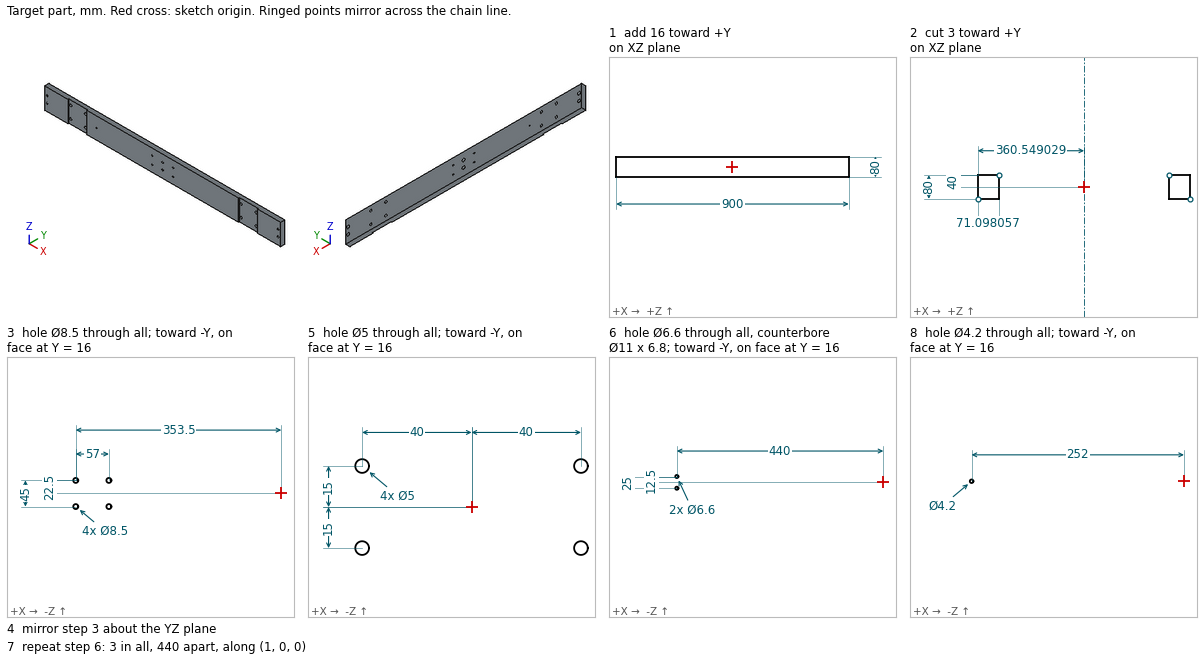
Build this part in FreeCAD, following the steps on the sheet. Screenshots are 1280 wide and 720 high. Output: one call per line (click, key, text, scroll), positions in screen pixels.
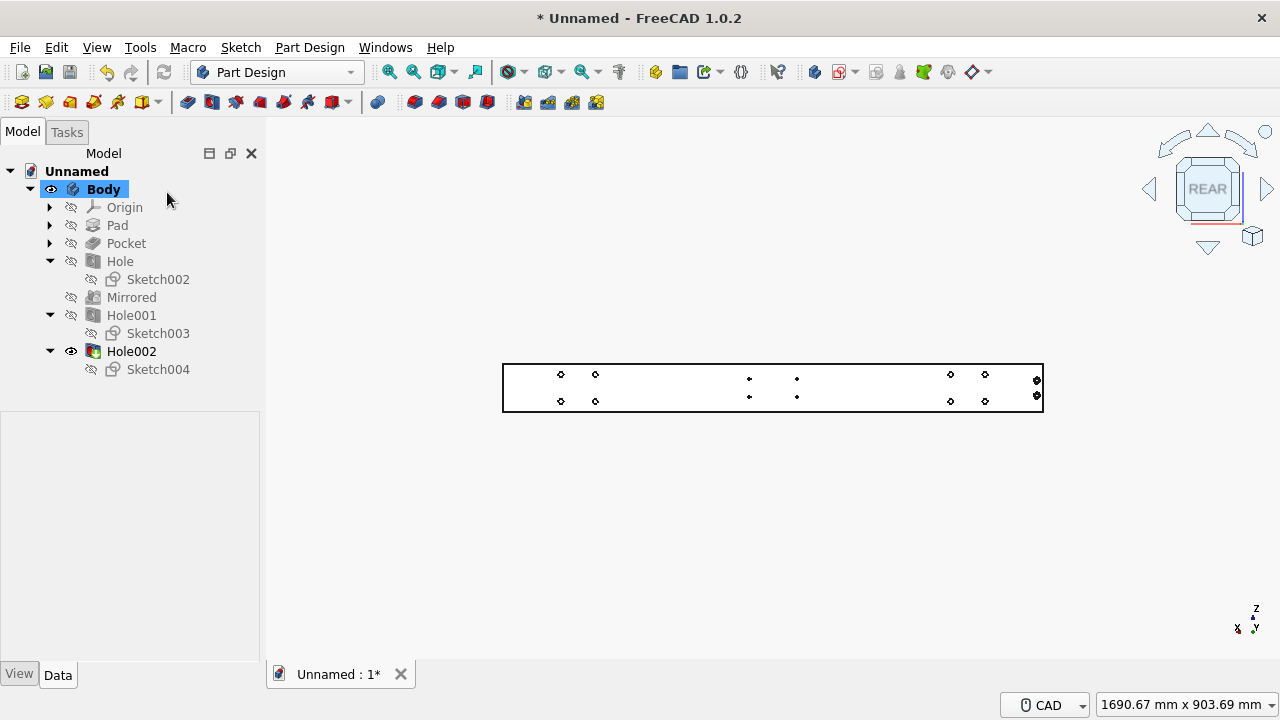
click(116, 351)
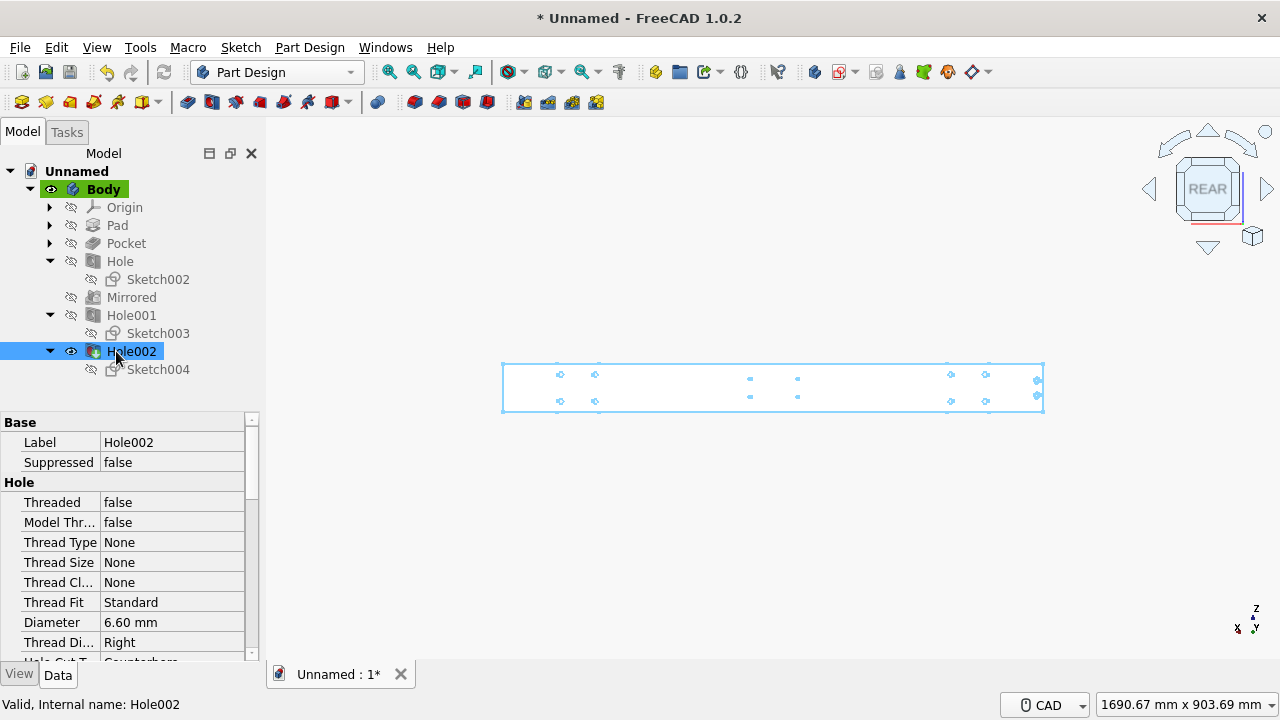
click(548, 102)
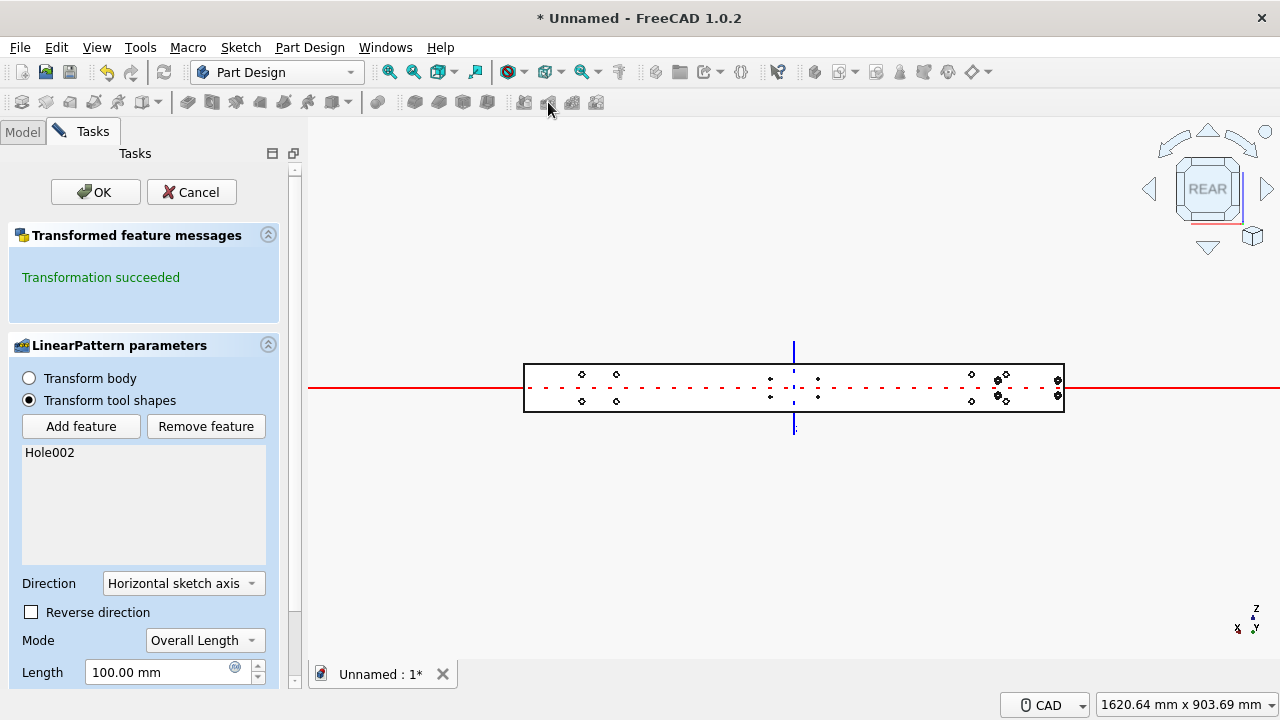
click(184, 584)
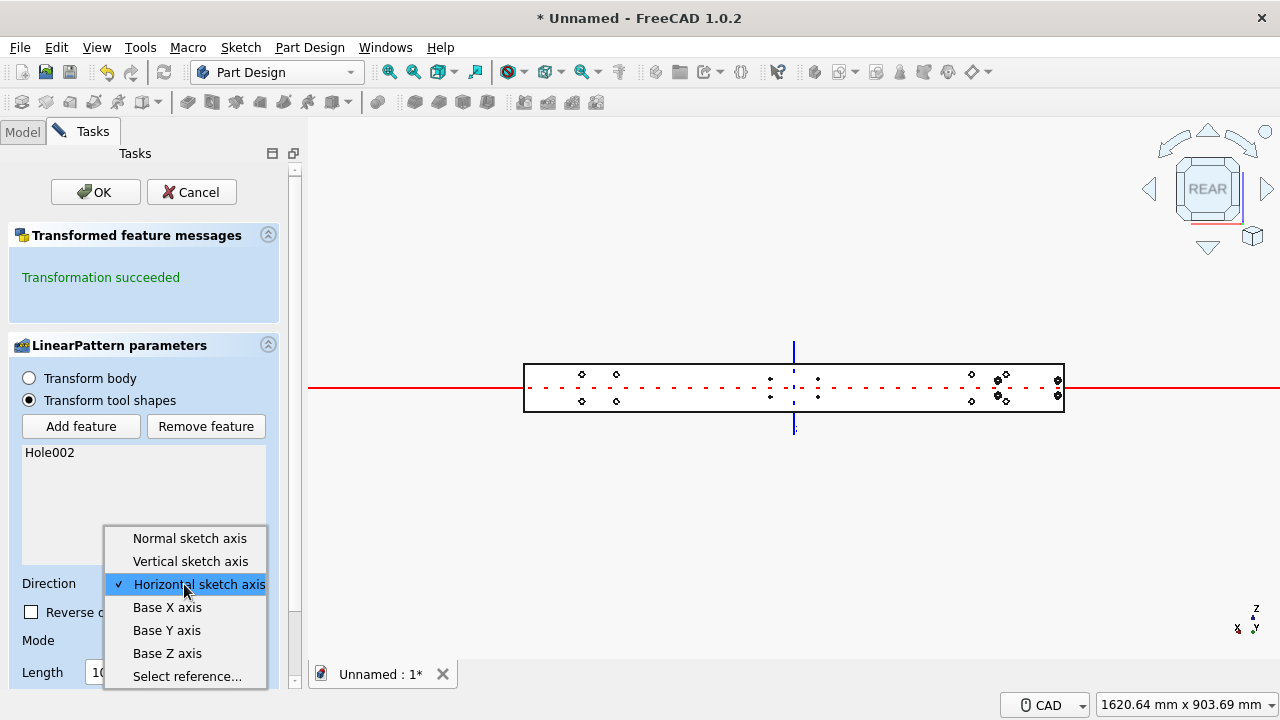
click(184, 608)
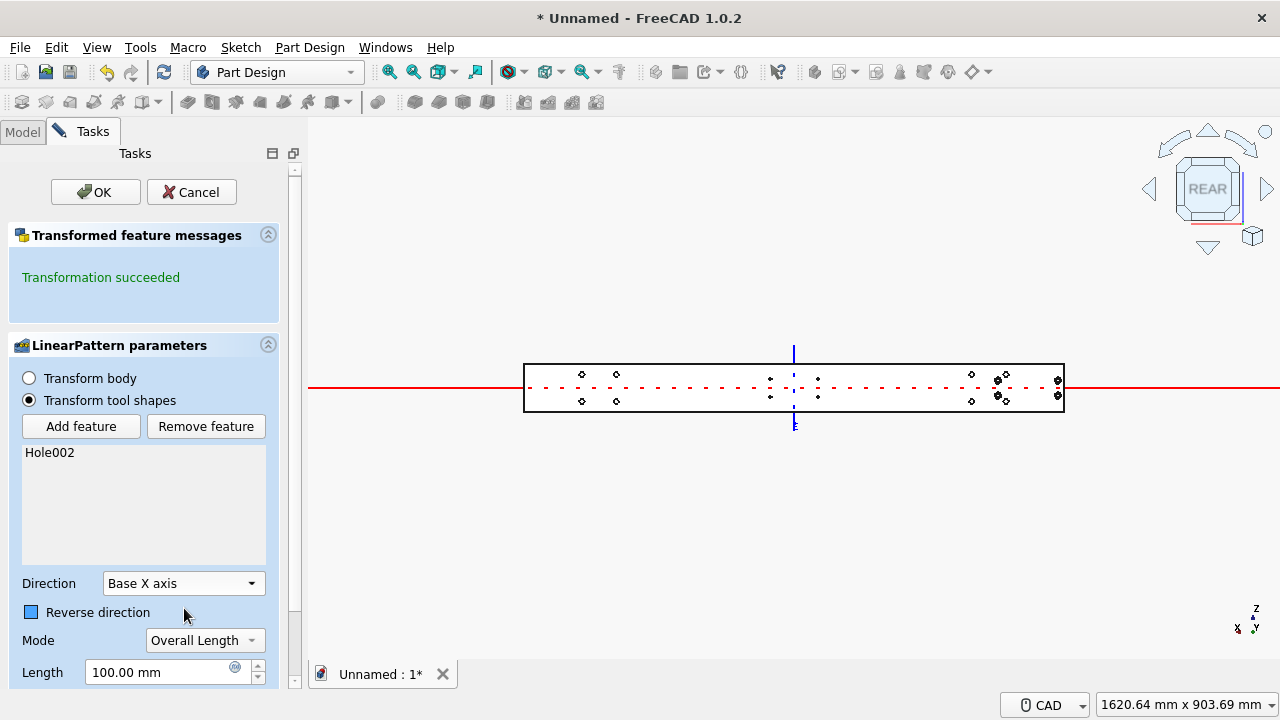
click(206, 640)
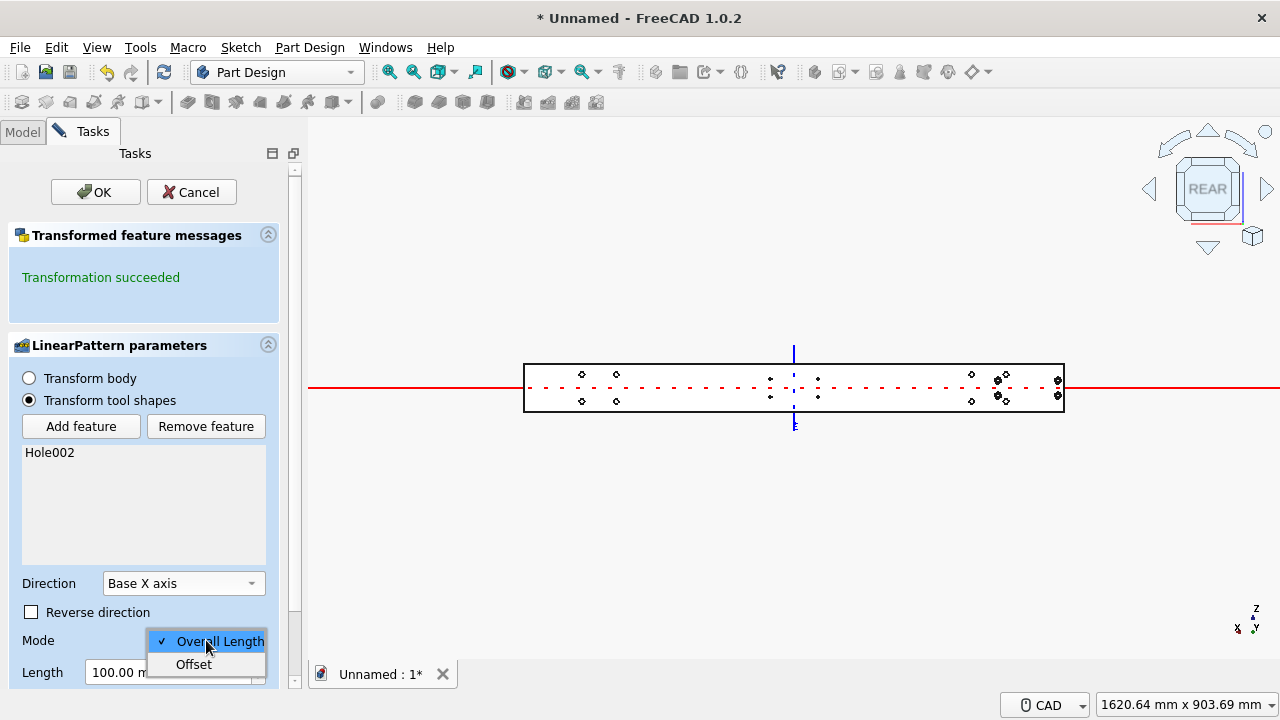
click(206, 664)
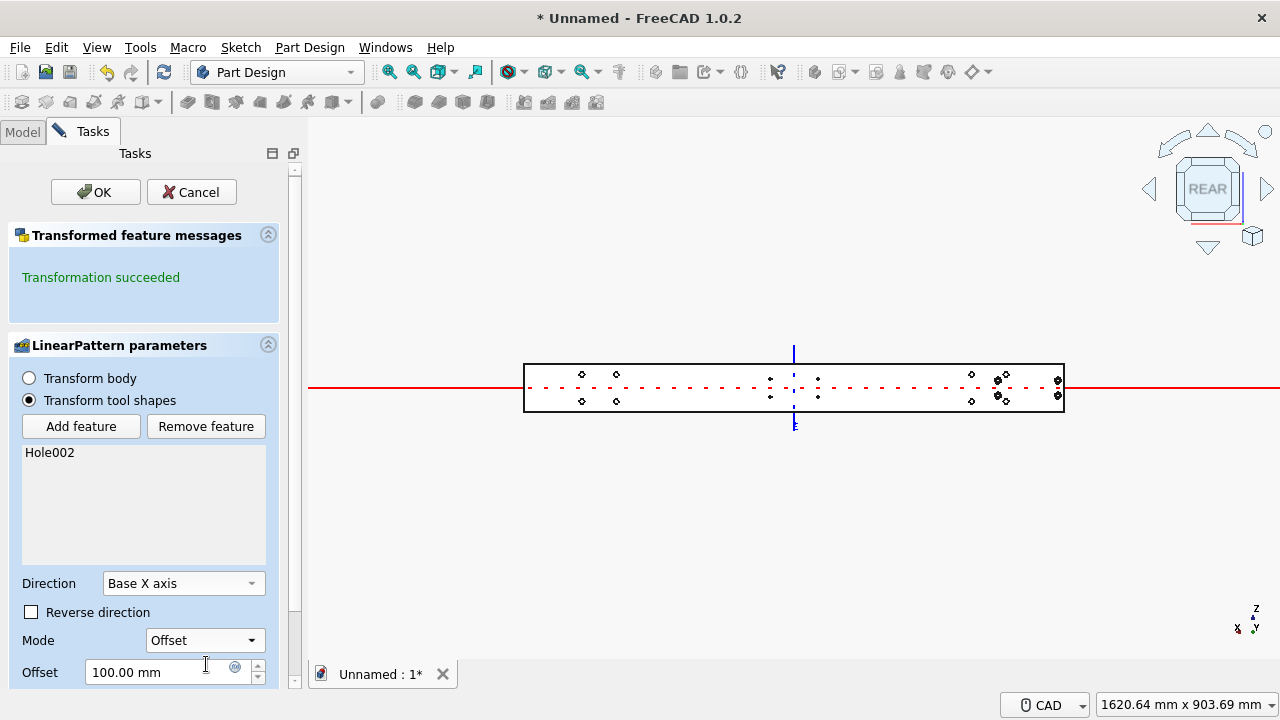
triple_click(168, 672)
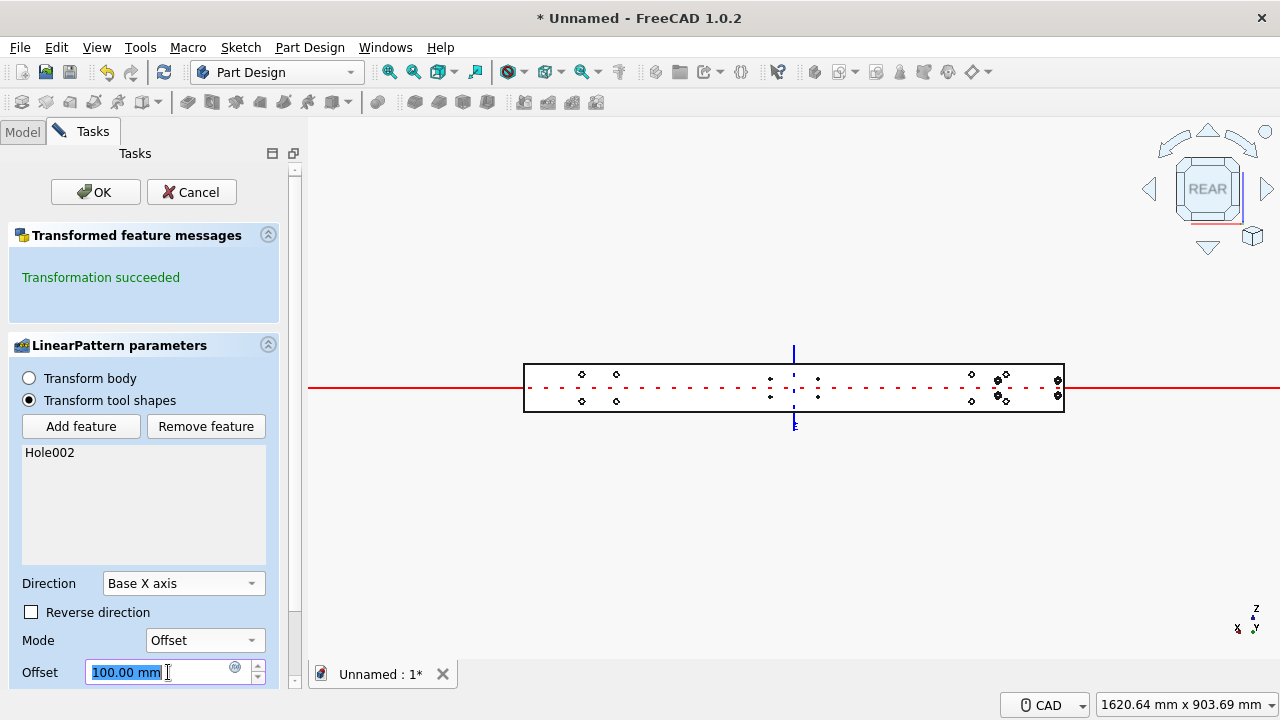
text(440)
key(Tab)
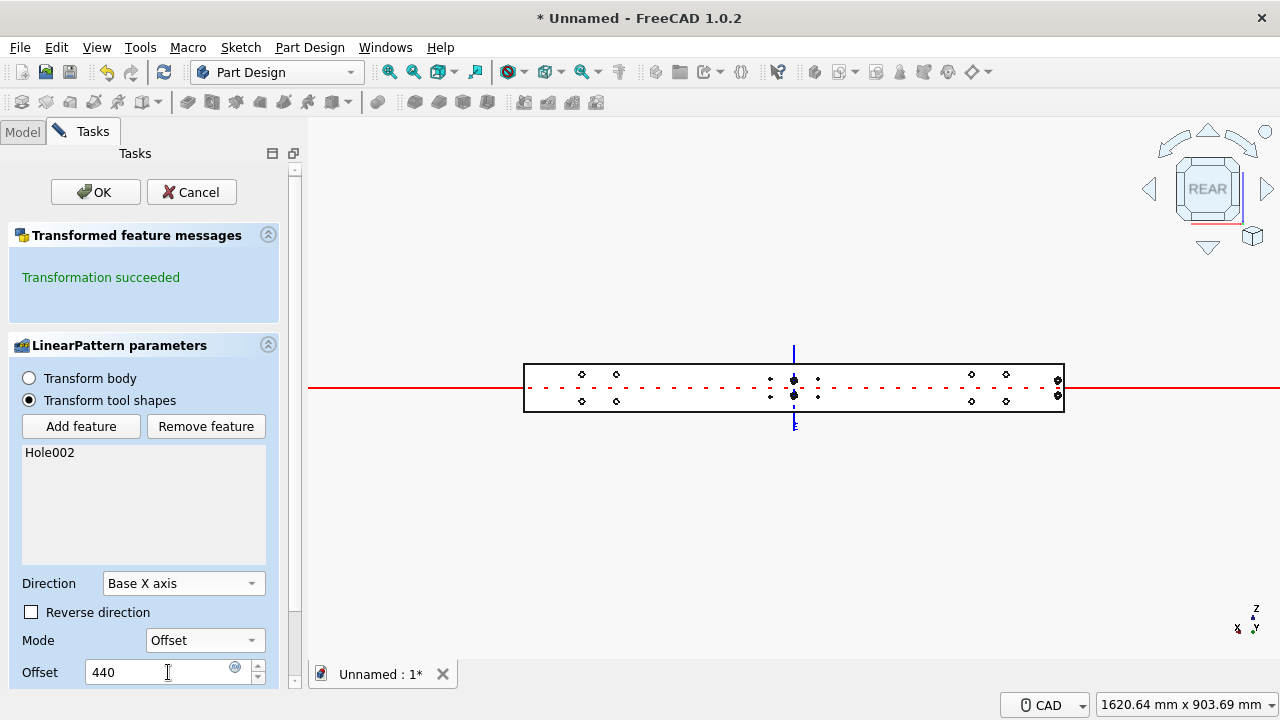
scroll(295, 426, down, 2)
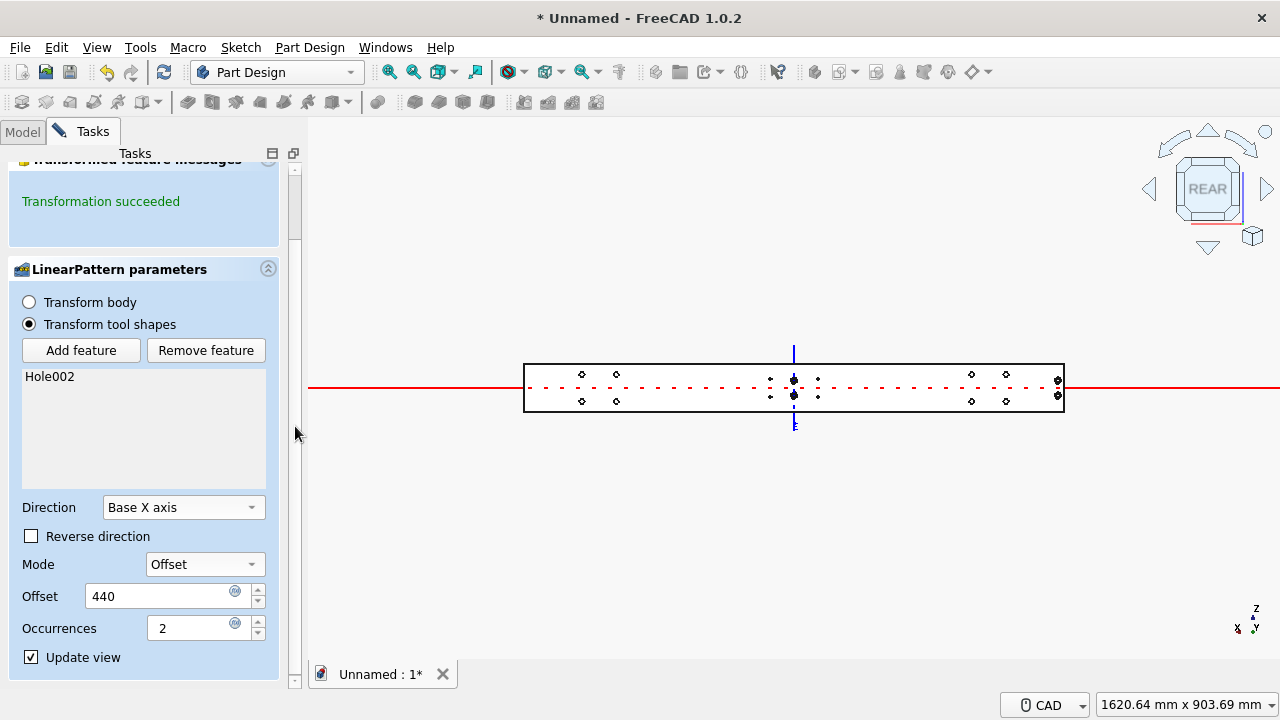
triple_click(198, 628)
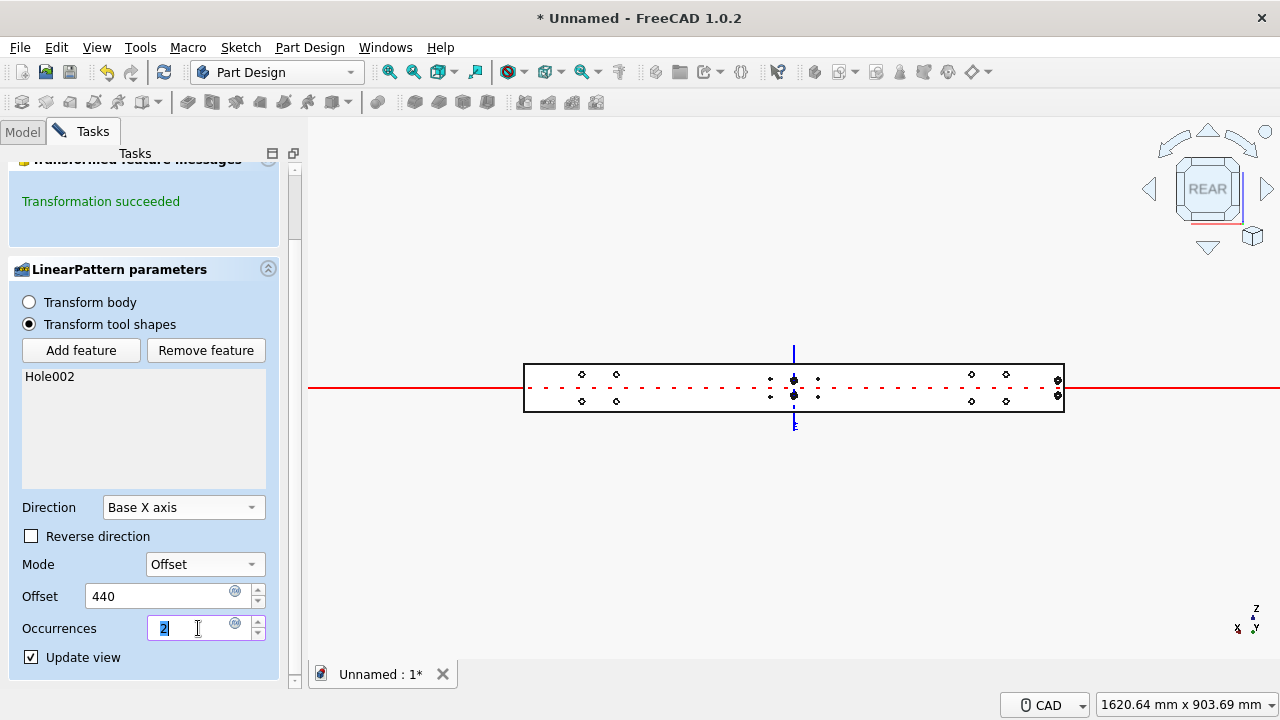
text(3)
key(Tab)